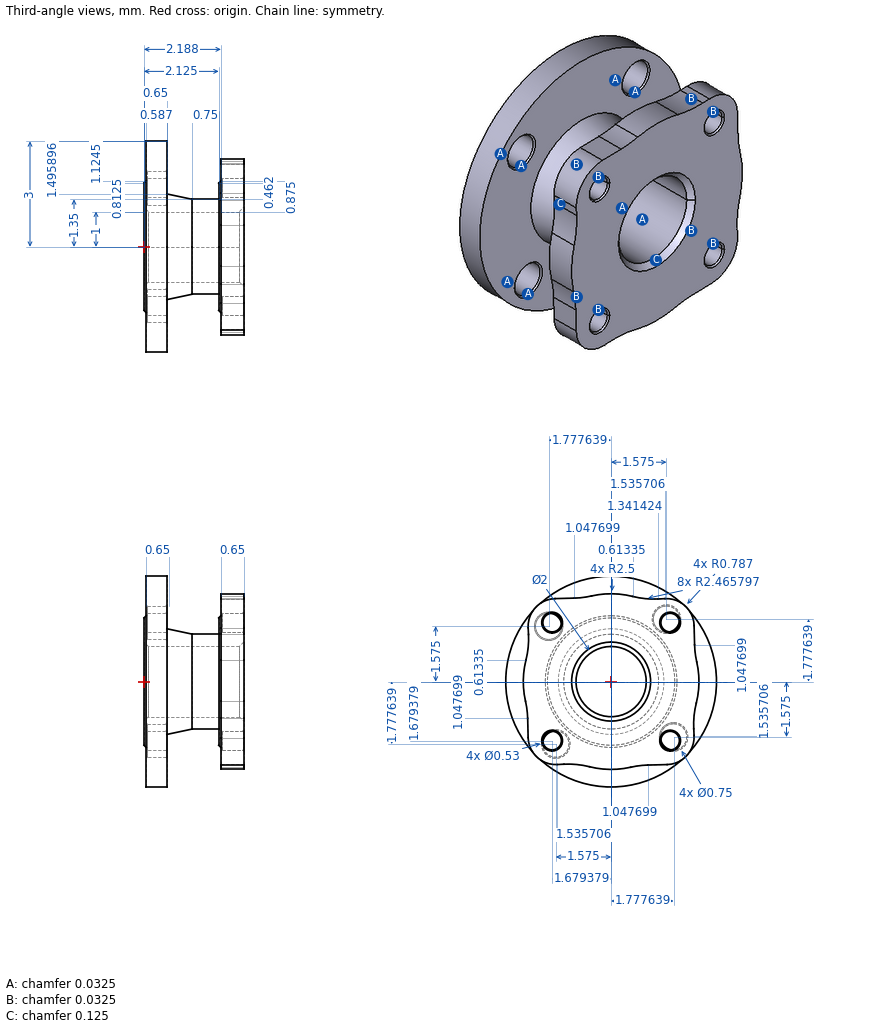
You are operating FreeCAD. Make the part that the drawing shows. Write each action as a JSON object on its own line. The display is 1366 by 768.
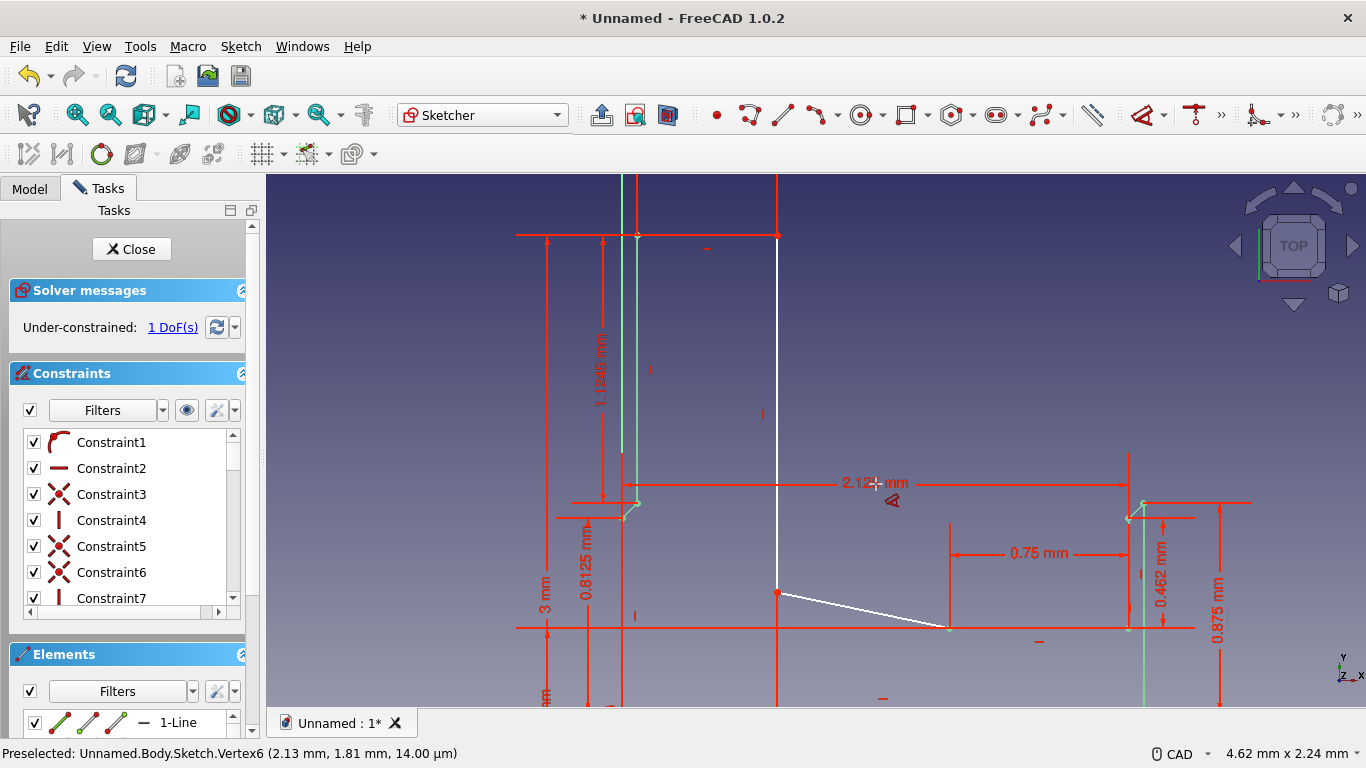
{"action": "left_click", "coordinate": [777, 485]}
{"action": "left_click", "coordinate": [743, 414]}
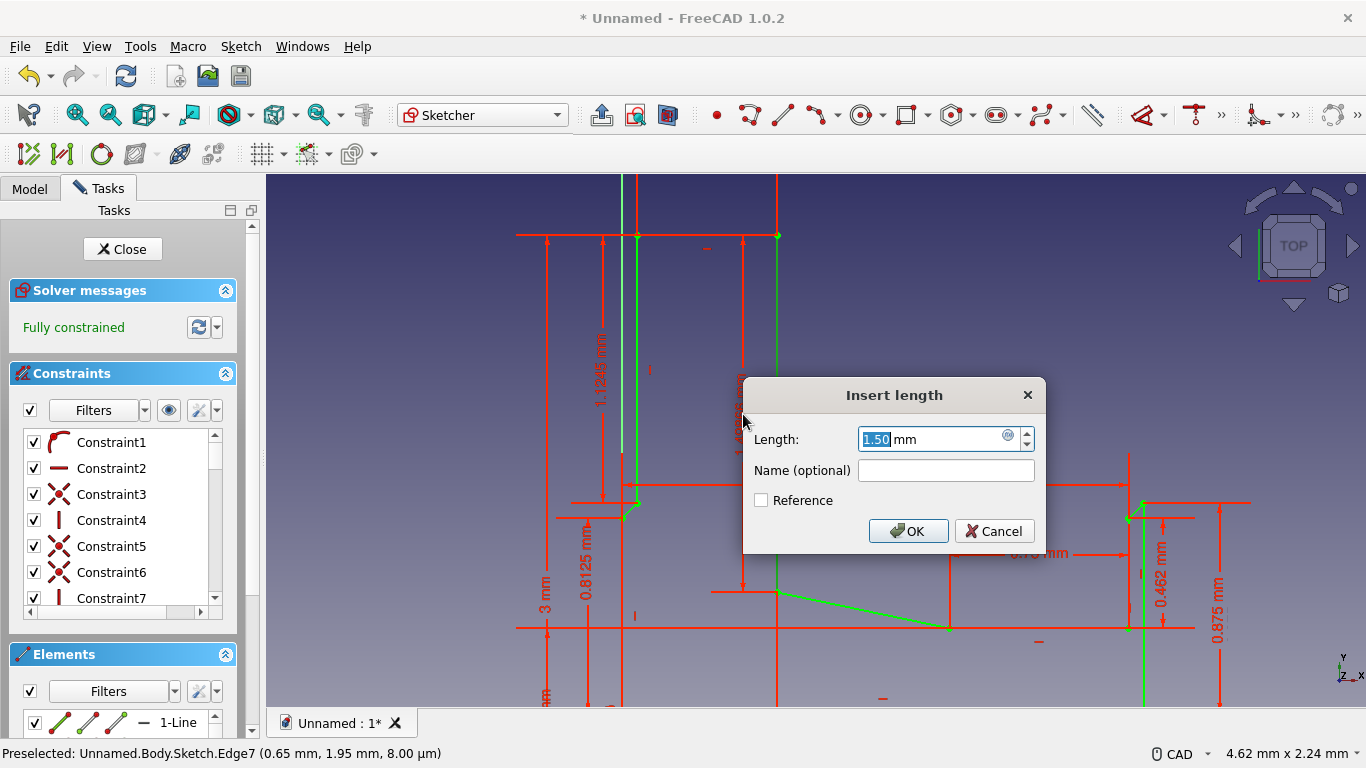
{"action": "type", "text": "1.495896"}
{"action": "key", "text": "Return"}
{"action": "key", "text": "Escape"}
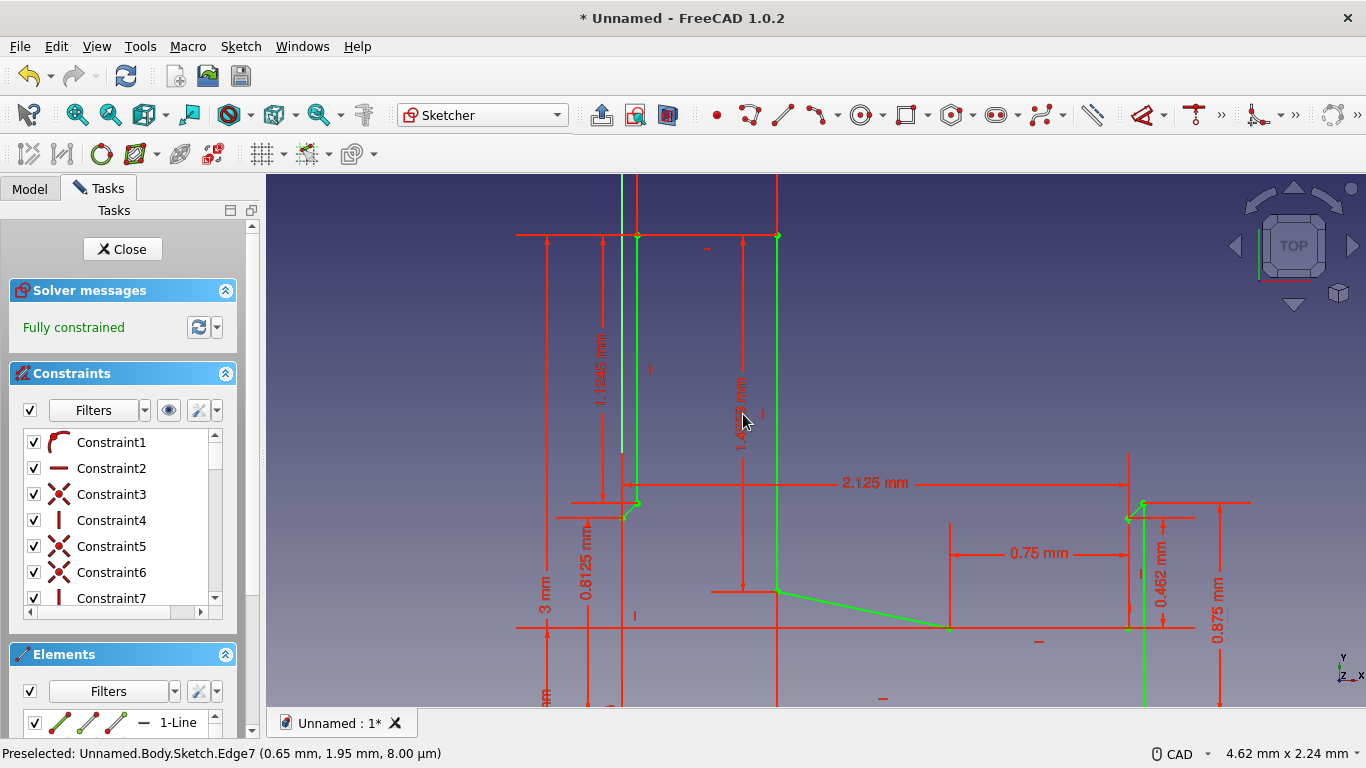
{"action": "left_click", "coordinate": [123, 249]}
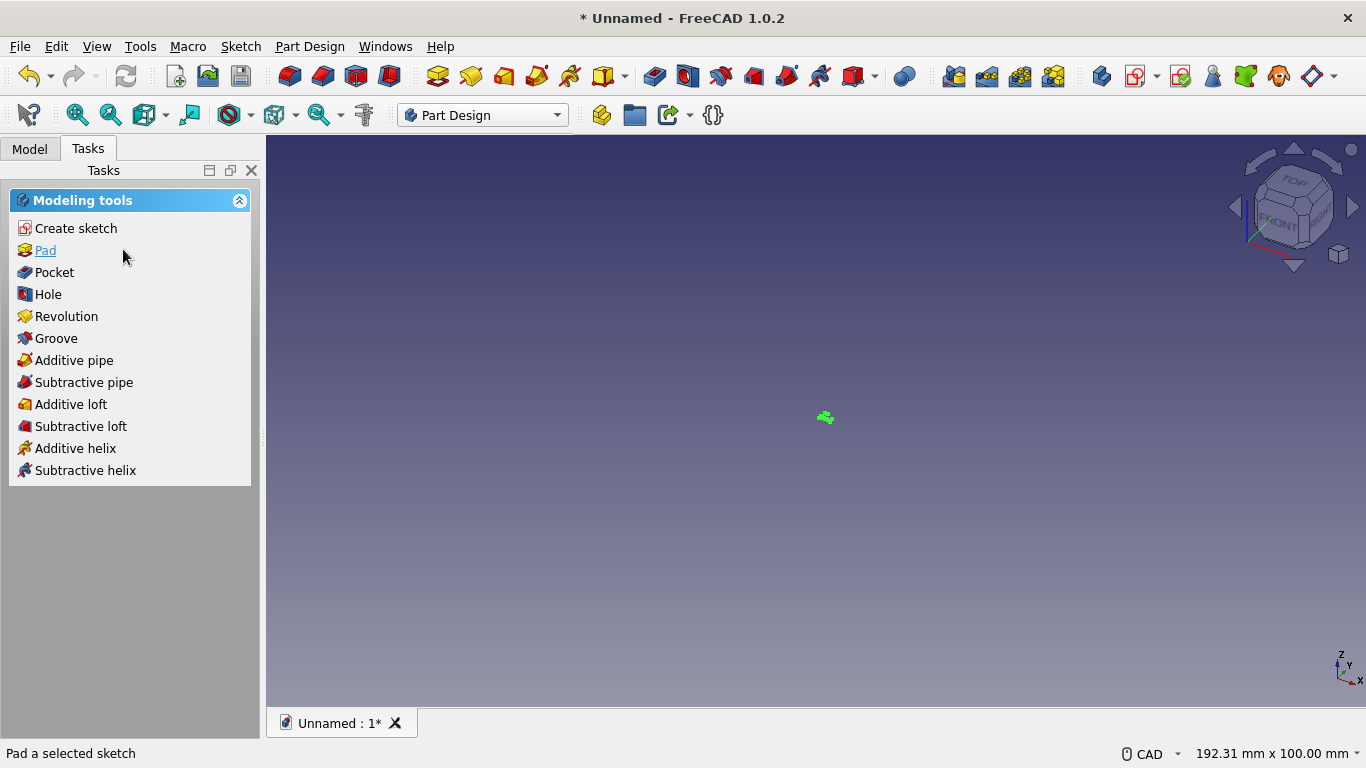
{"action": "left_click", "coordinate": [471, 76]}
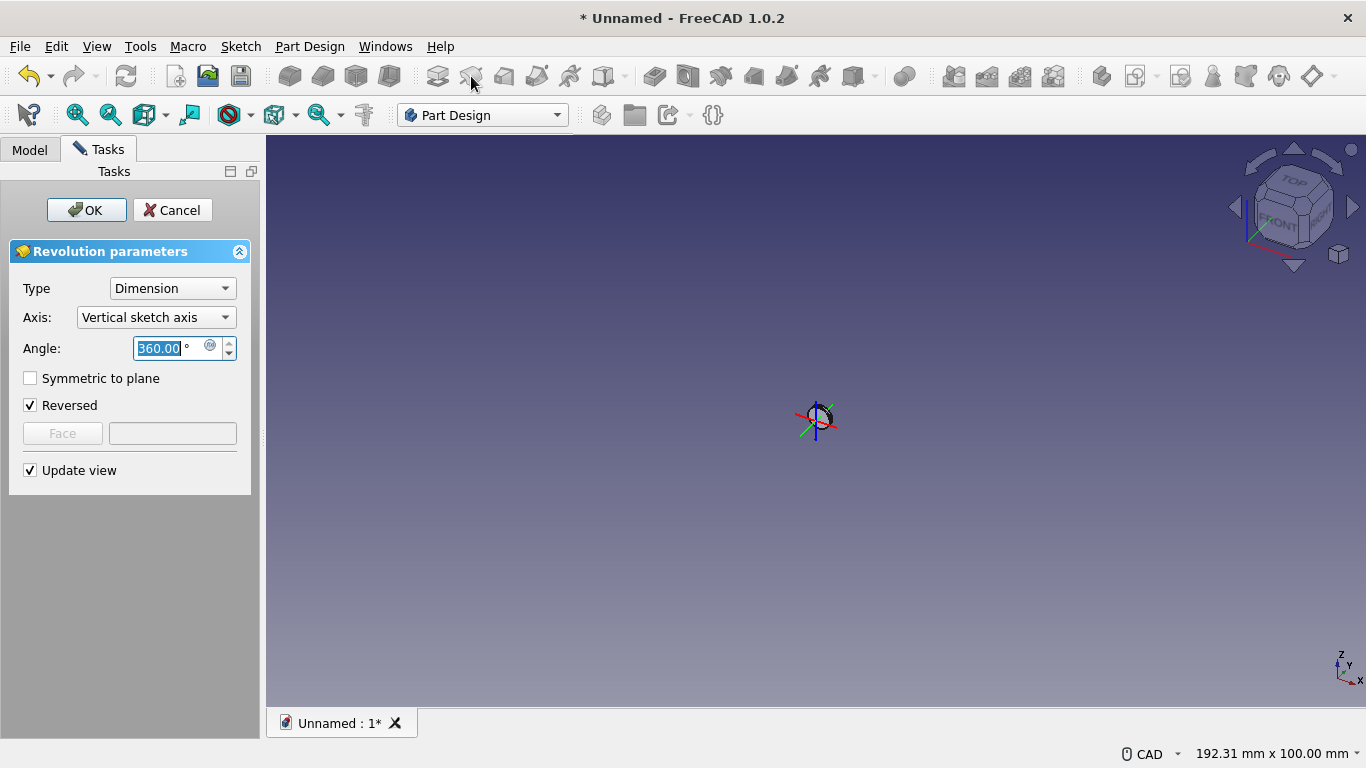
{"action": "left_click", "coordinate": [157, 318]}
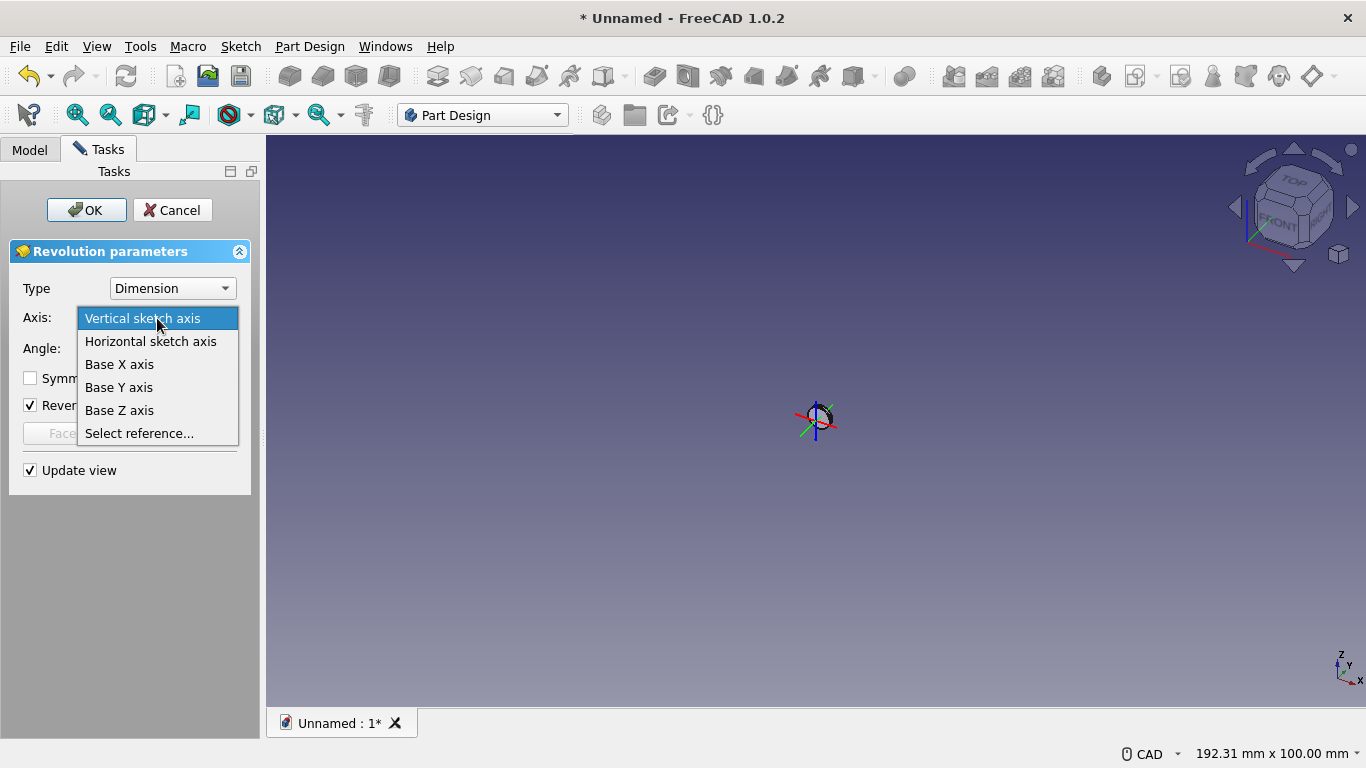
{"action": "left_click", "coordinate": [156, 342]}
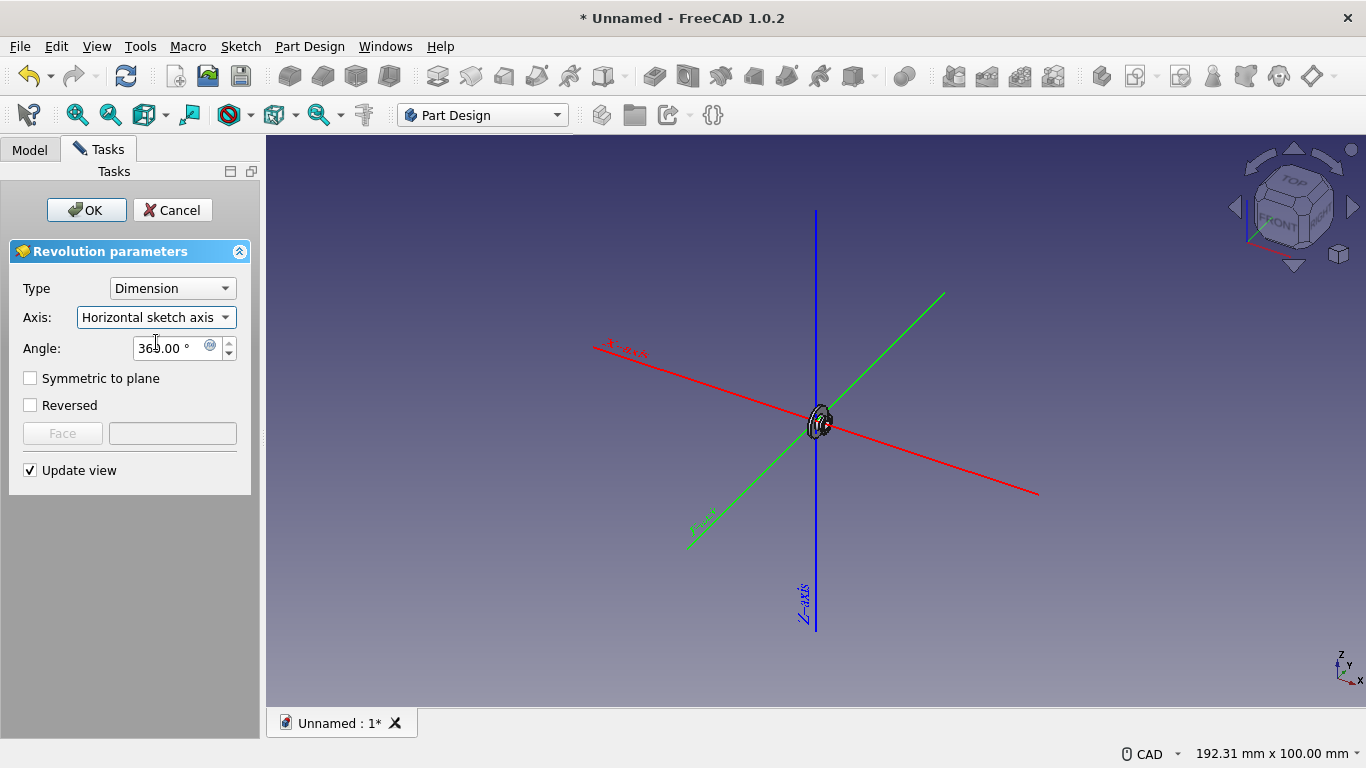
{"action": "left_click", "coordinate": [87, 210]}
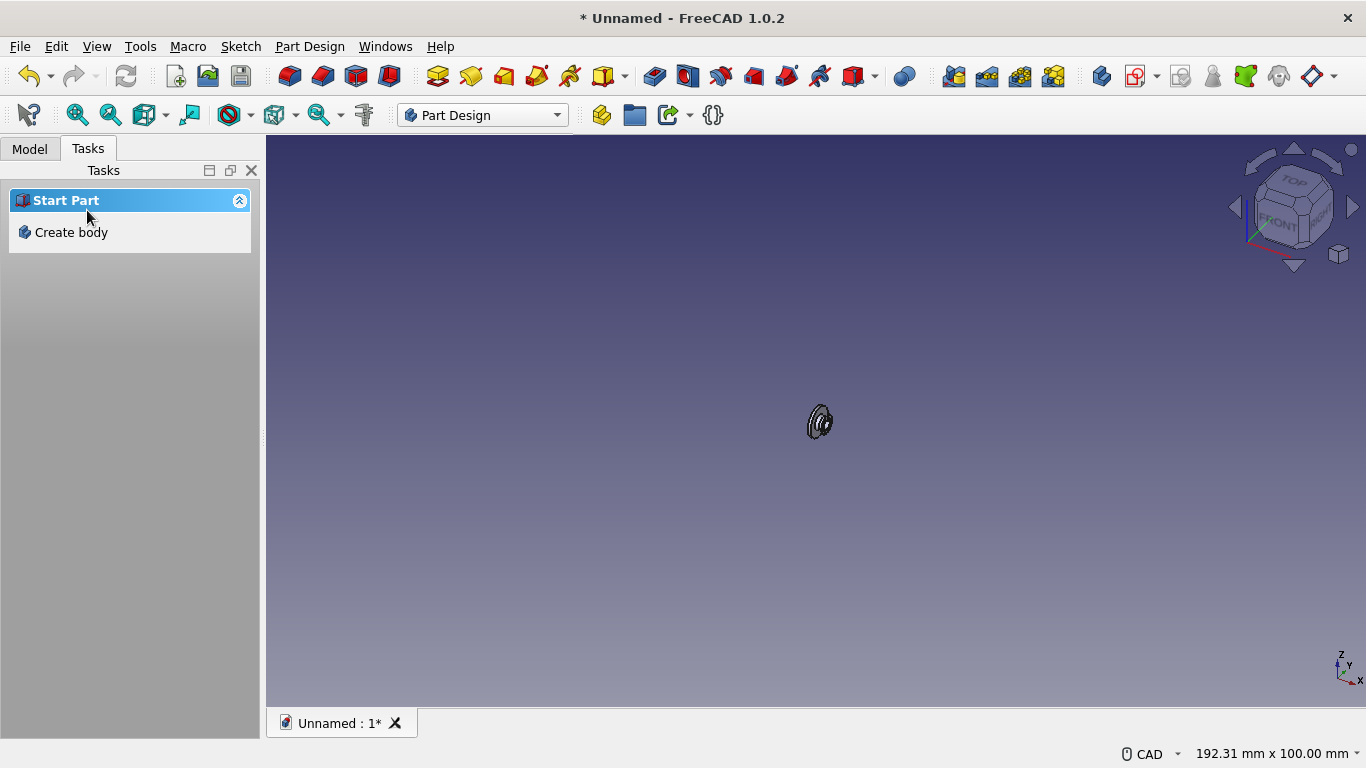
{"action": "left_click", "coordinate": [78, 116]}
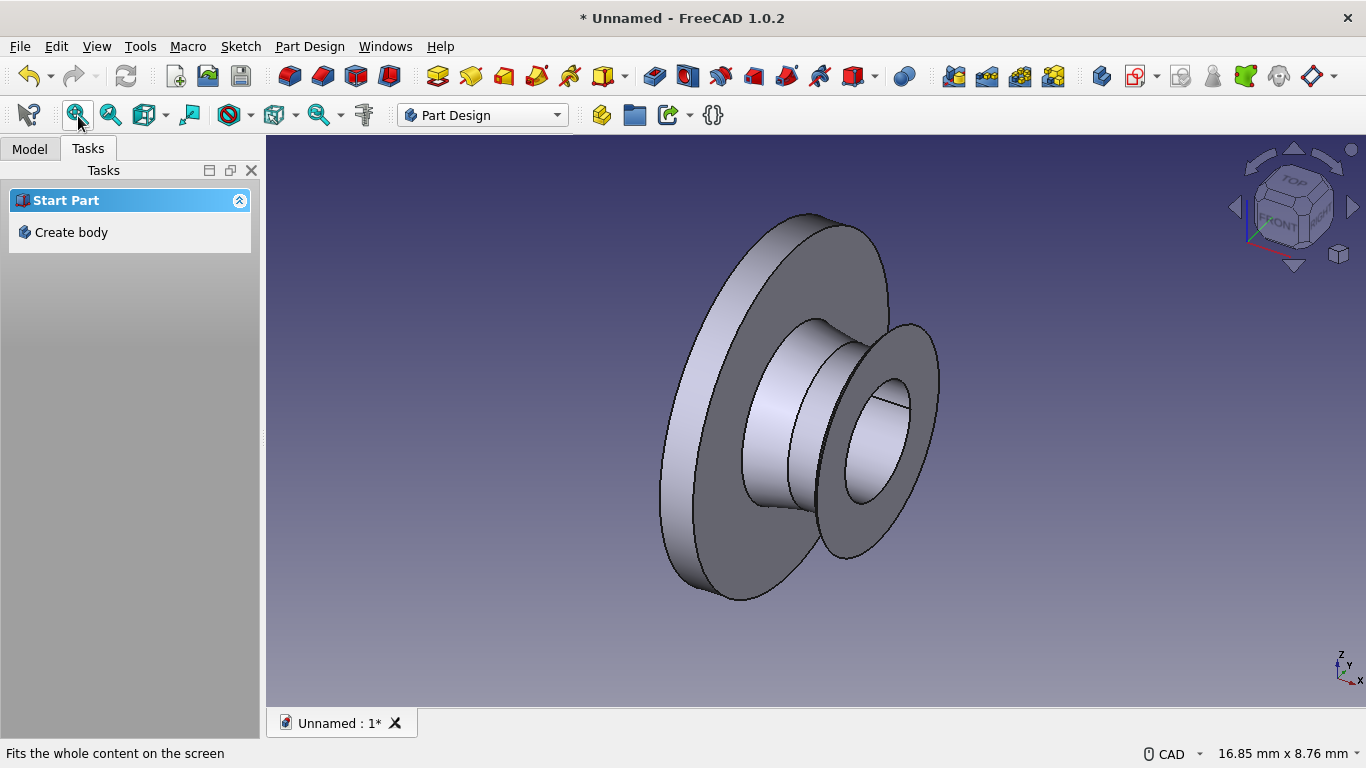
{"action": "left_click", "coordinate": [913, 348]}